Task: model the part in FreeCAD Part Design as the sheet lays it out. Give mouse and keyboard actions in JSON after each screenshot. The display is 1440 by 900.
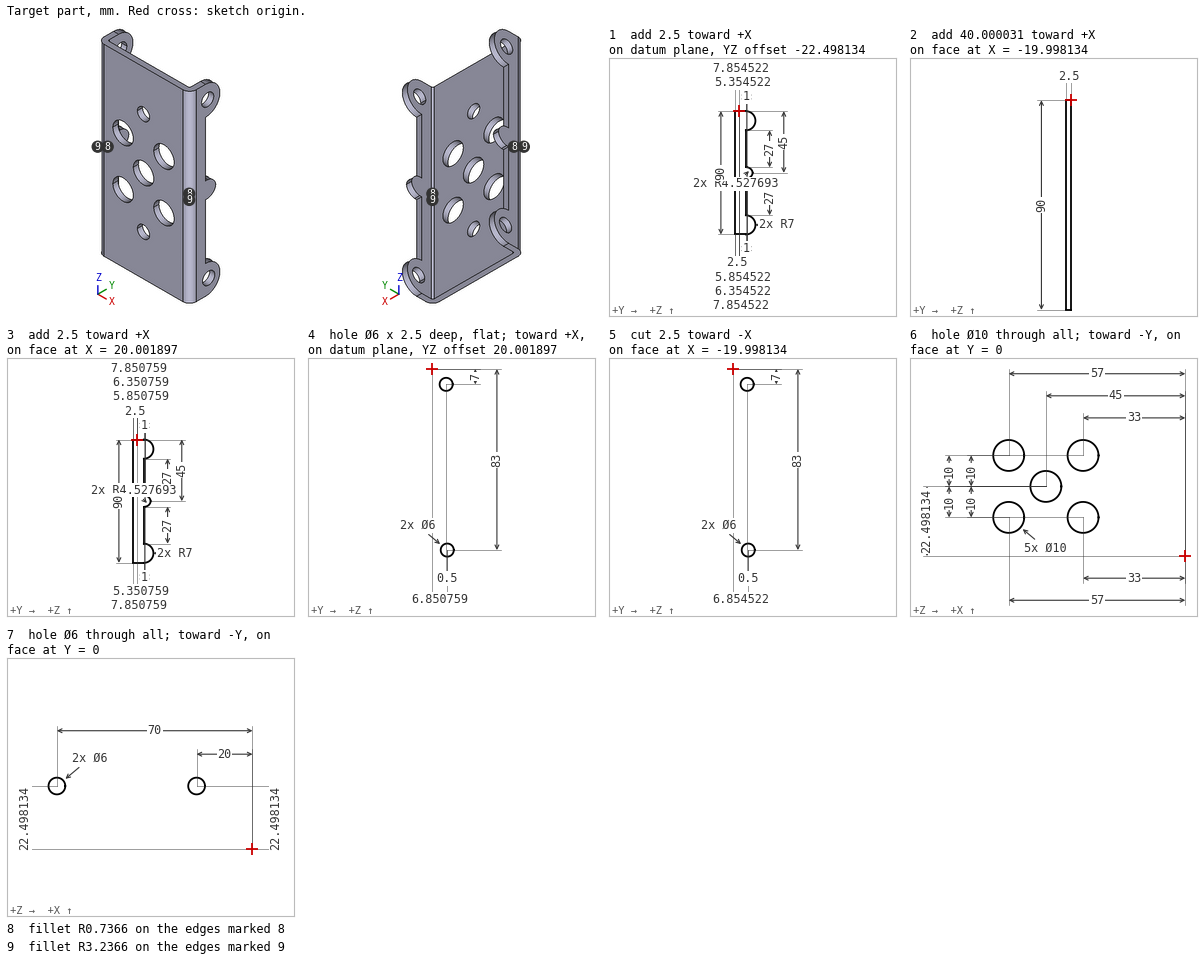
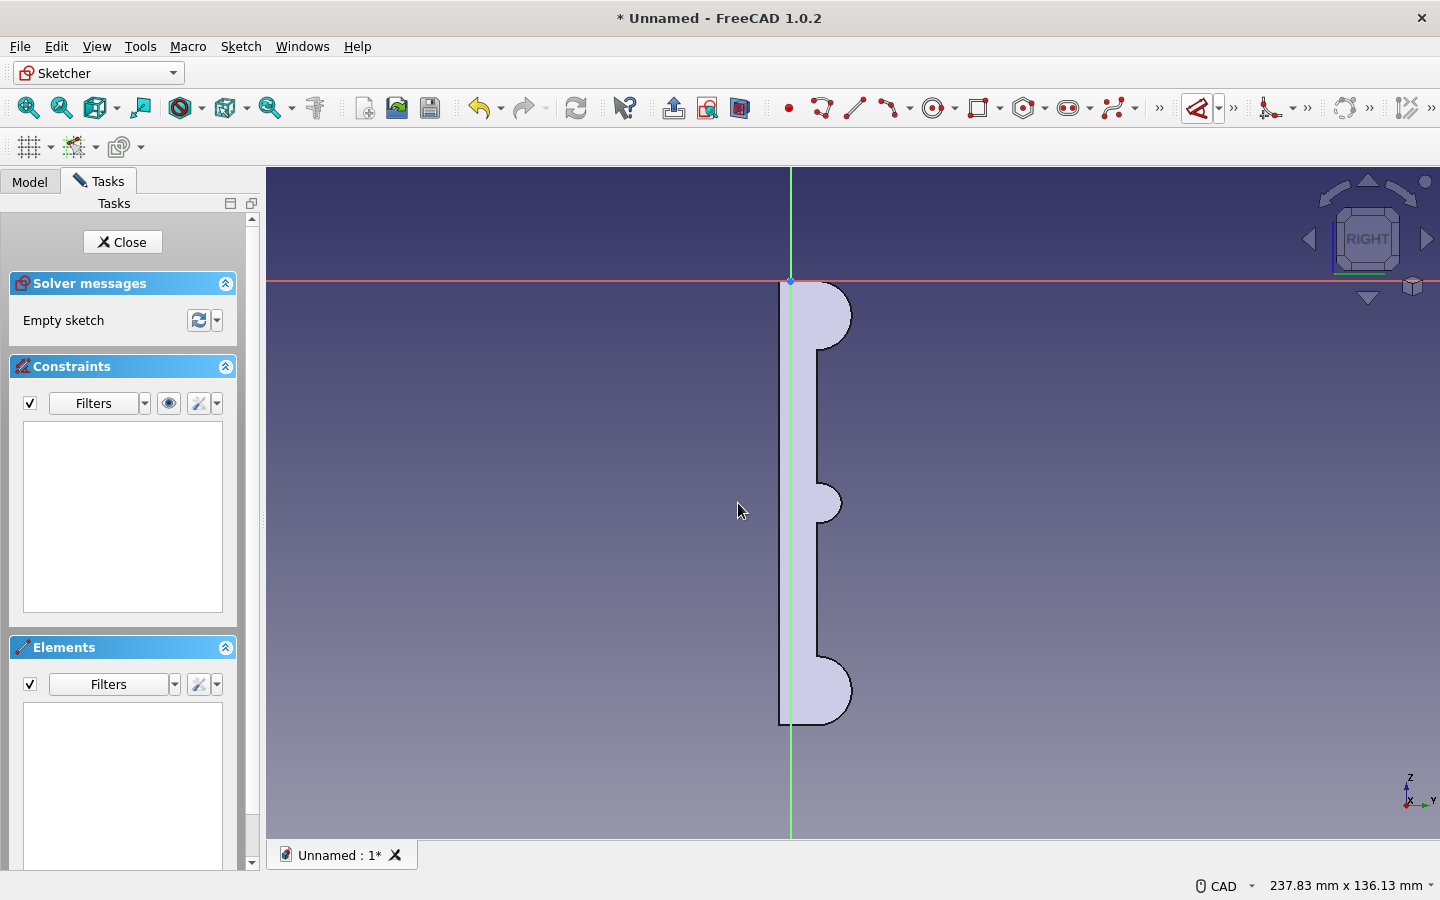
{"action": "left_click", "coordinate": [978, 108]}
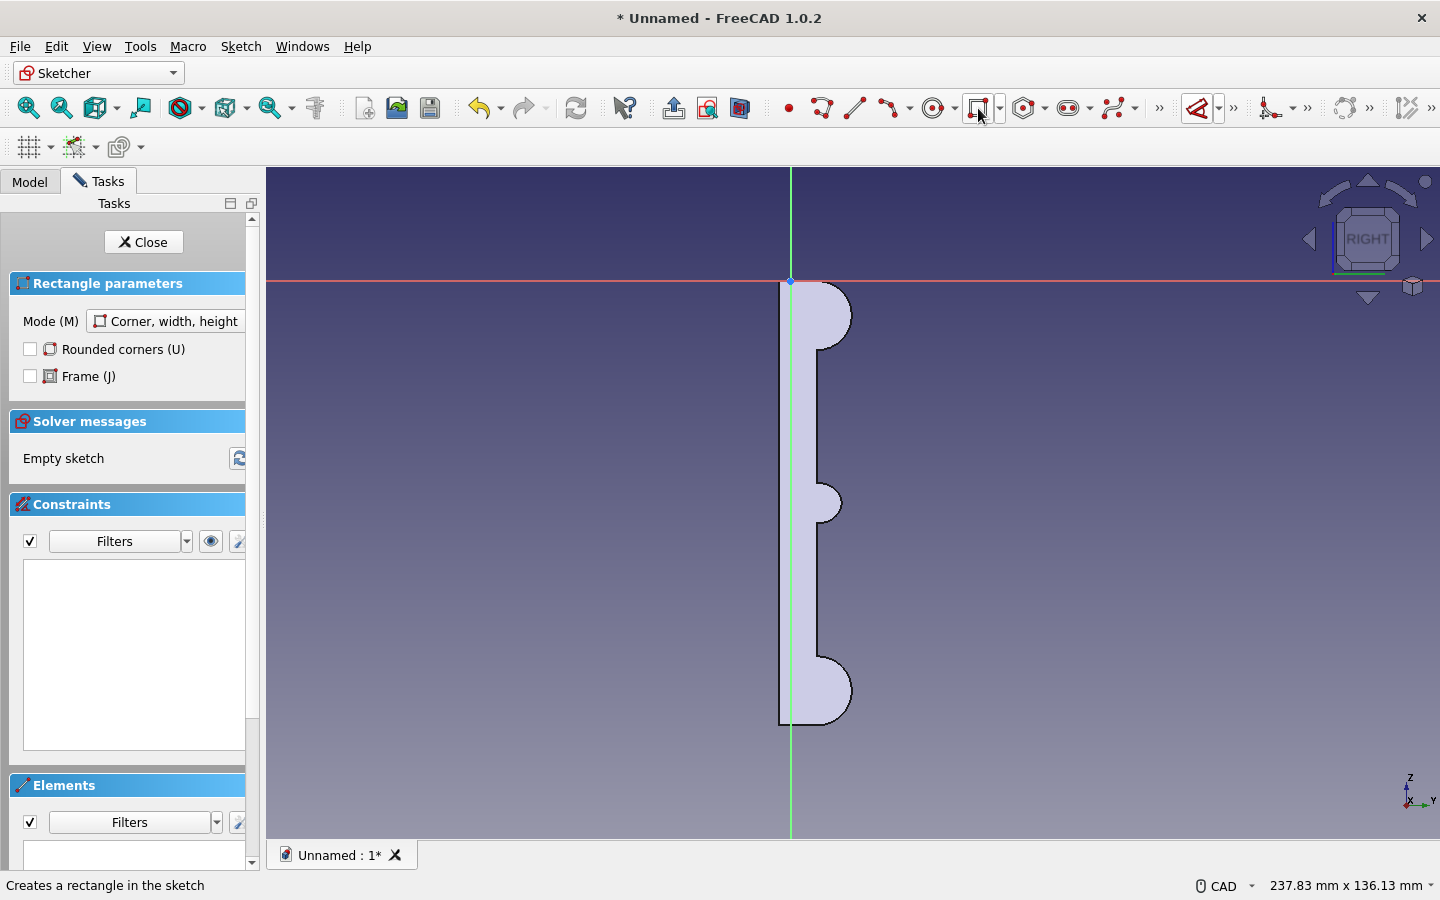
{"action": "scroll", "coordinate": [791, 281], "scroll_direction": "up", "scroll_amount": 2}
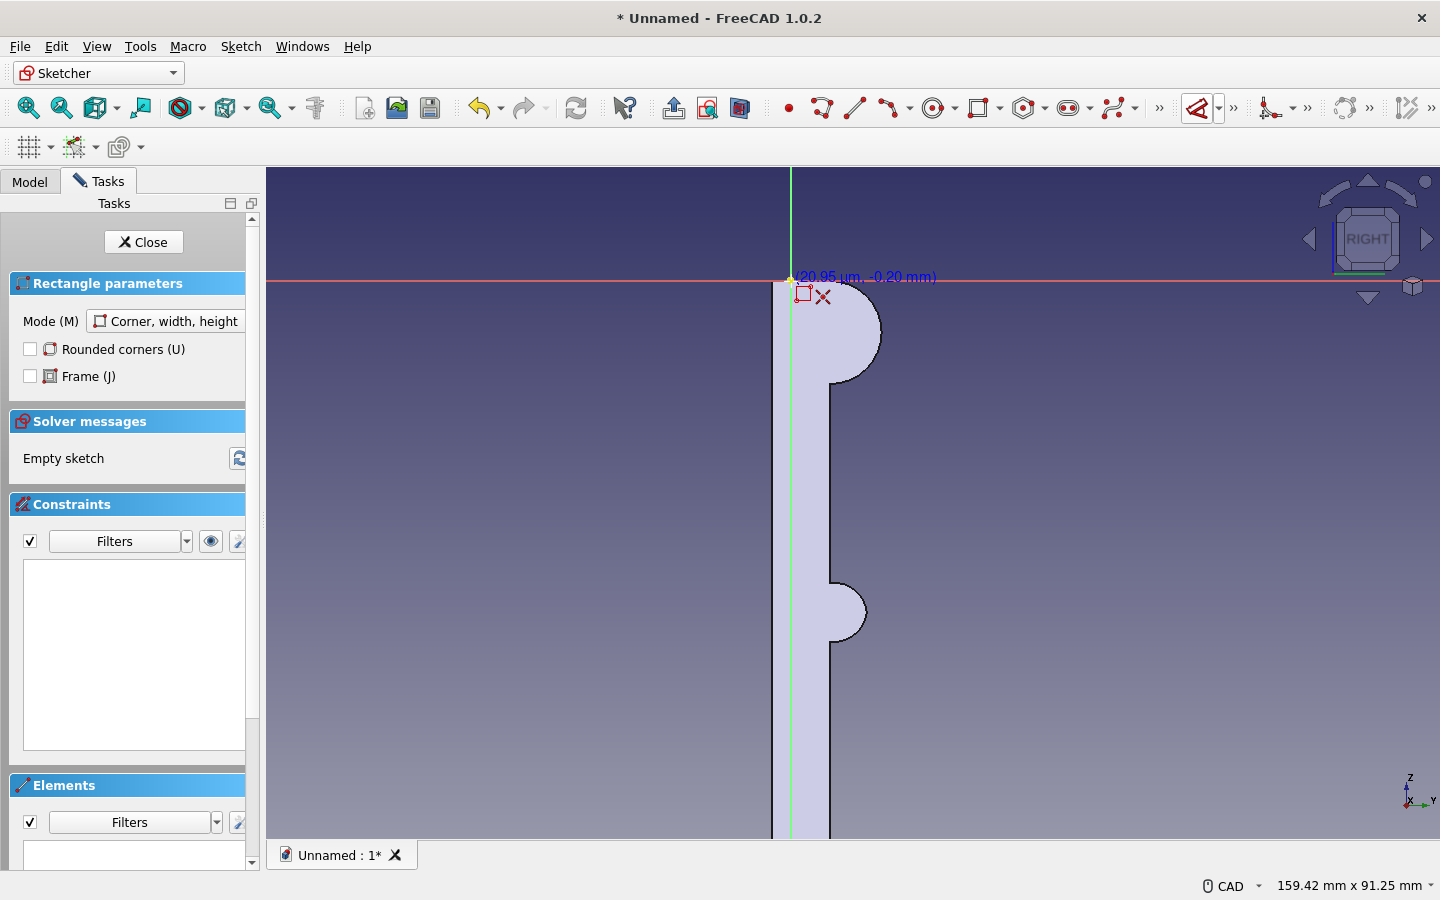
{"action": "left_click", "coordinate": [791, 281]}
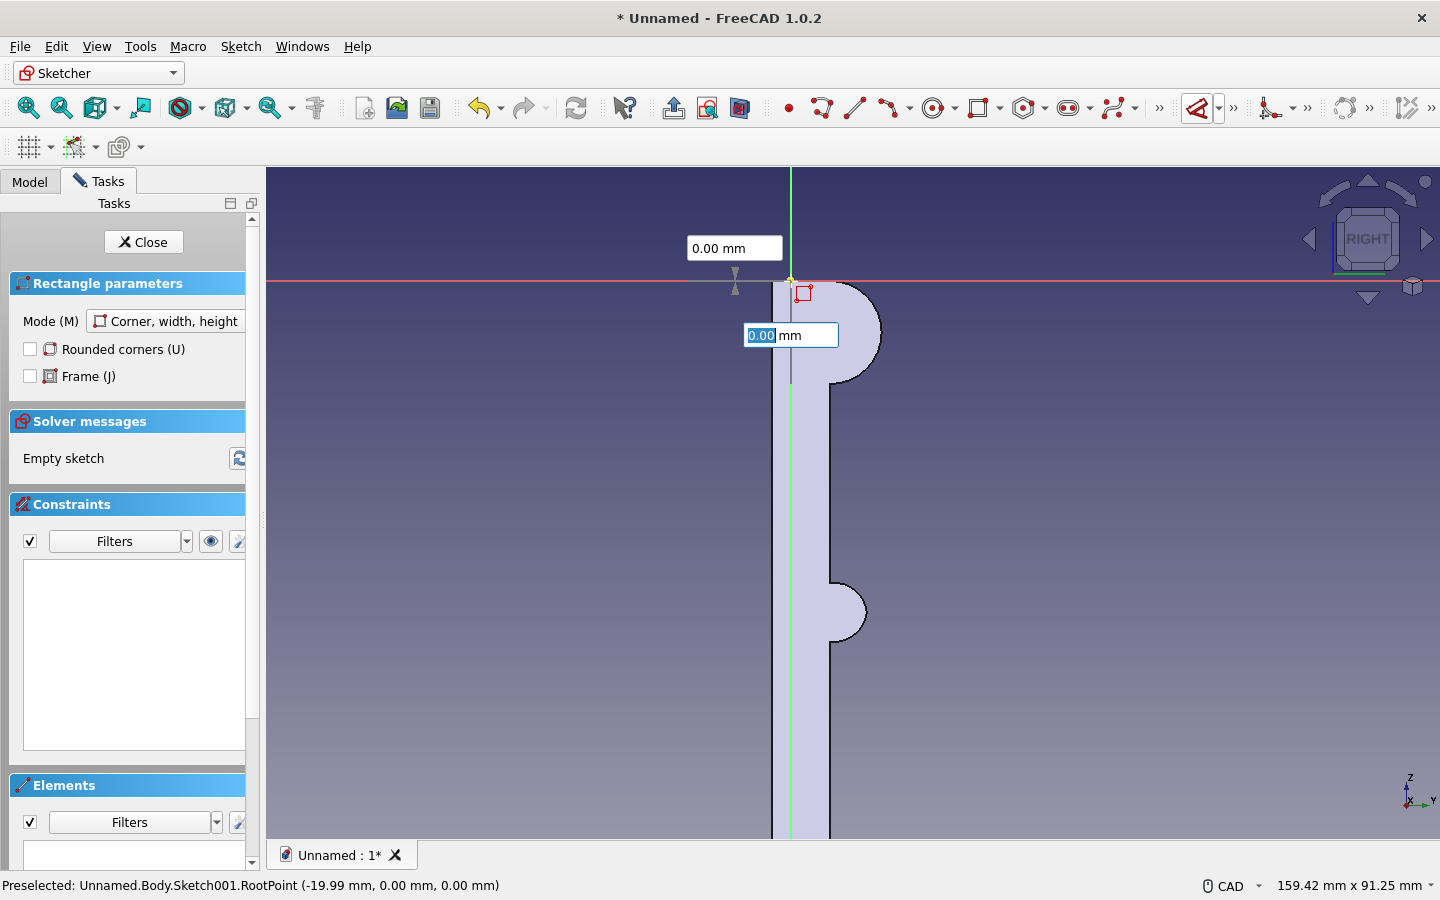
{"action": "scroll", "coordinate": [791, 281], "scroll_direction": "down", "scroll_amount": 2}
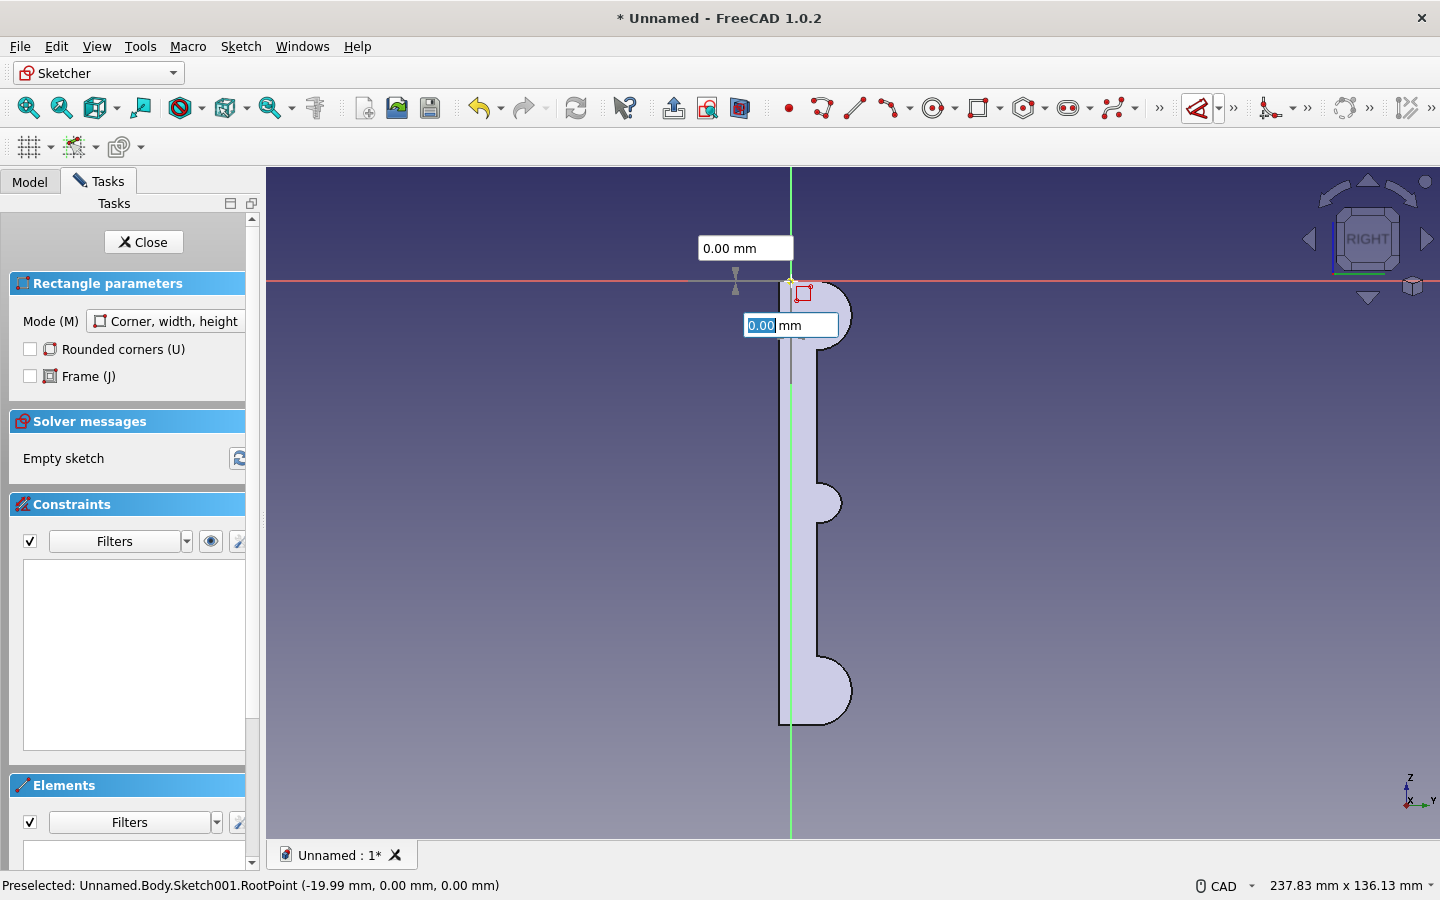
{"action": "scroll", "coordinate": [779, 725], "scroll_direction": "up", "scroll_amount": 2}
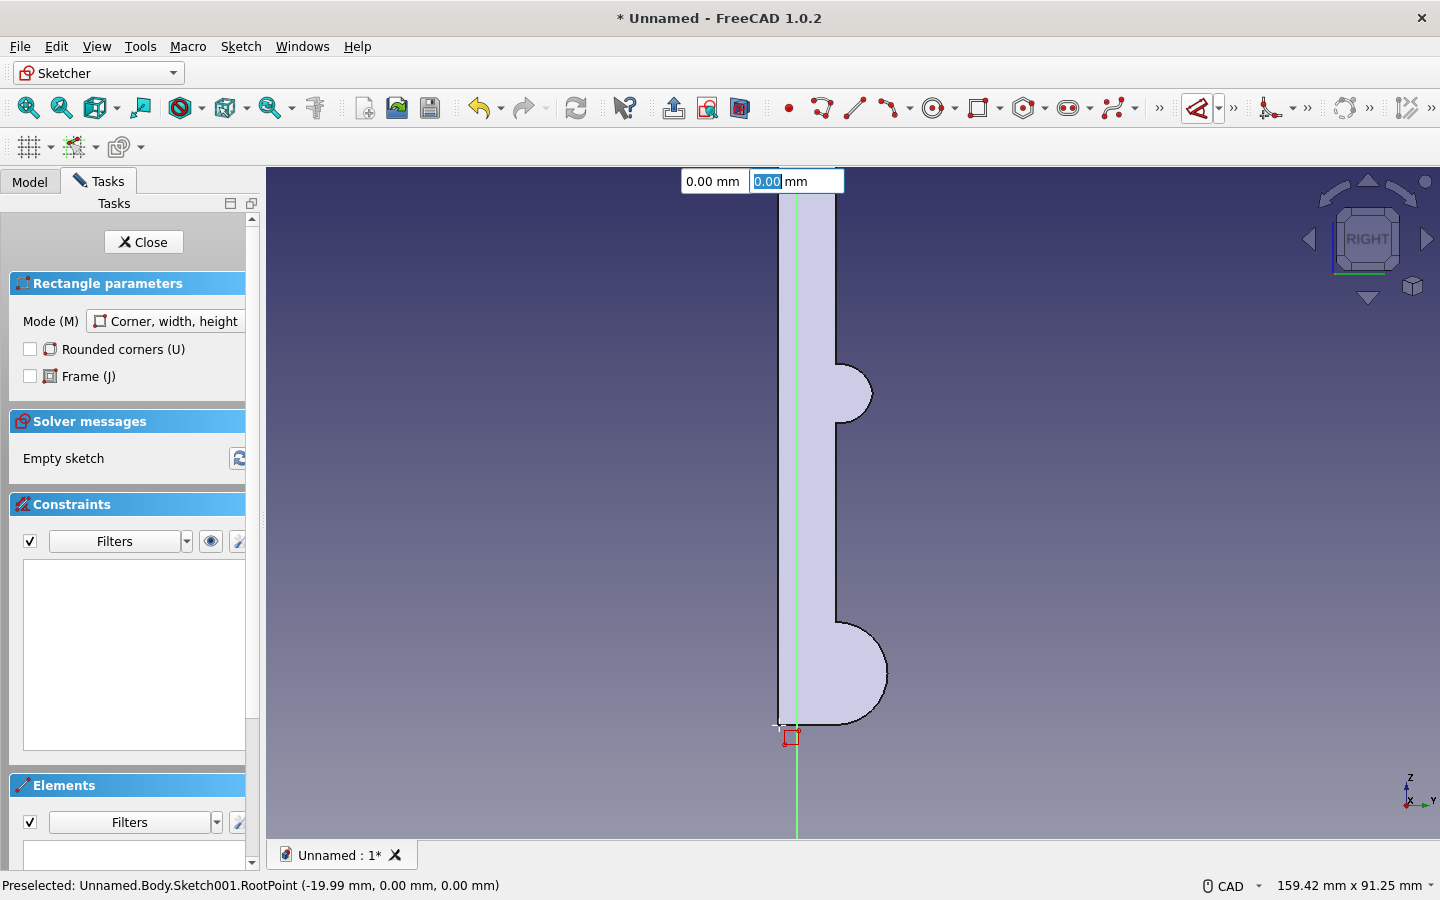
{"action": "left_click", "coordinate": [778, 725]}
{"action": "key", "text": "Escape"}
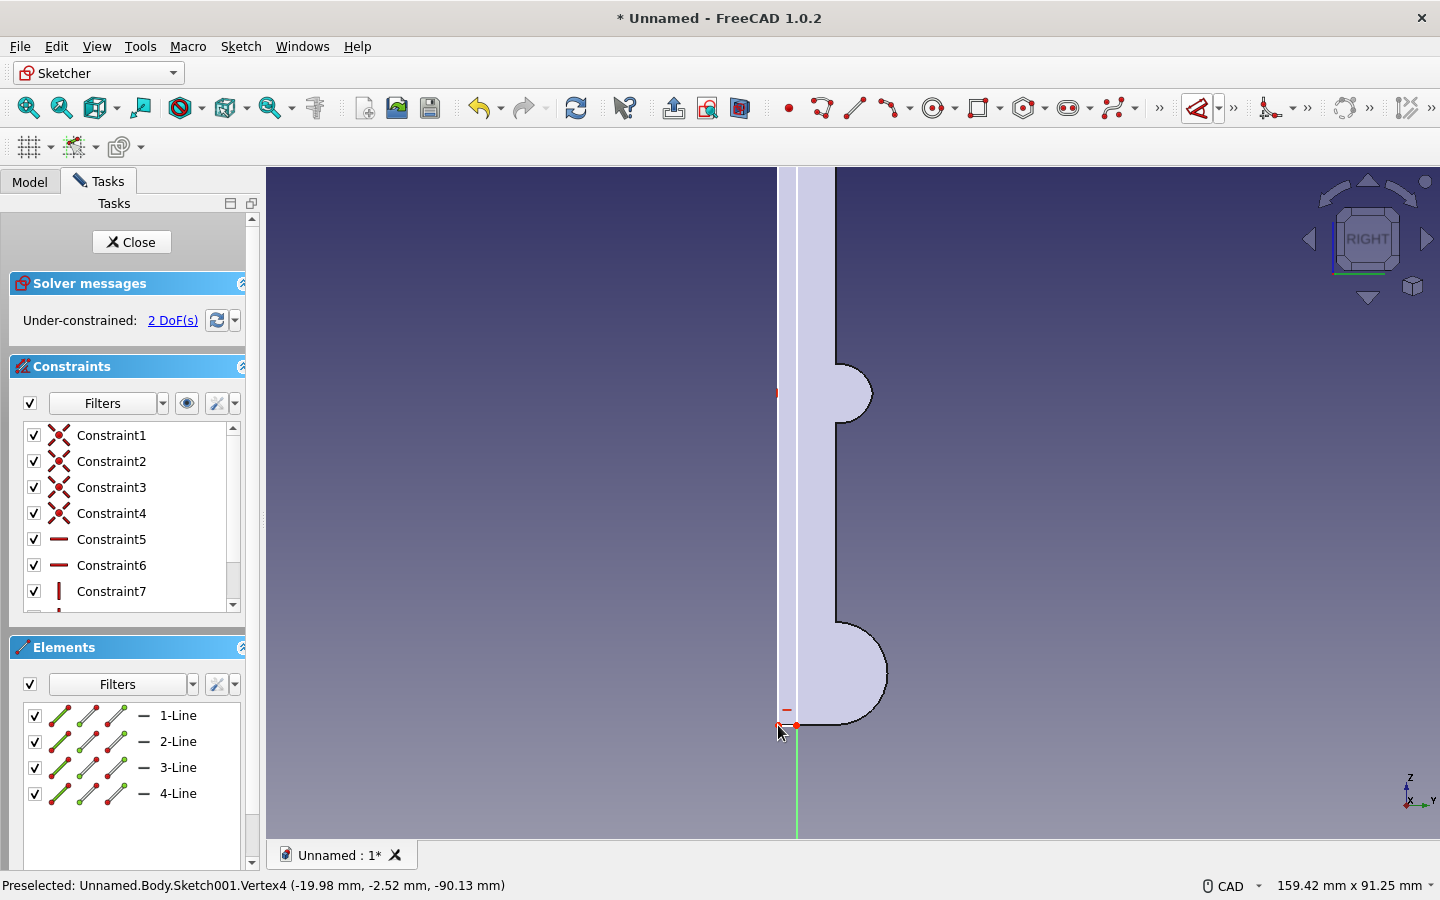
{"action": "left_click", "coordinate": [778, 261]}